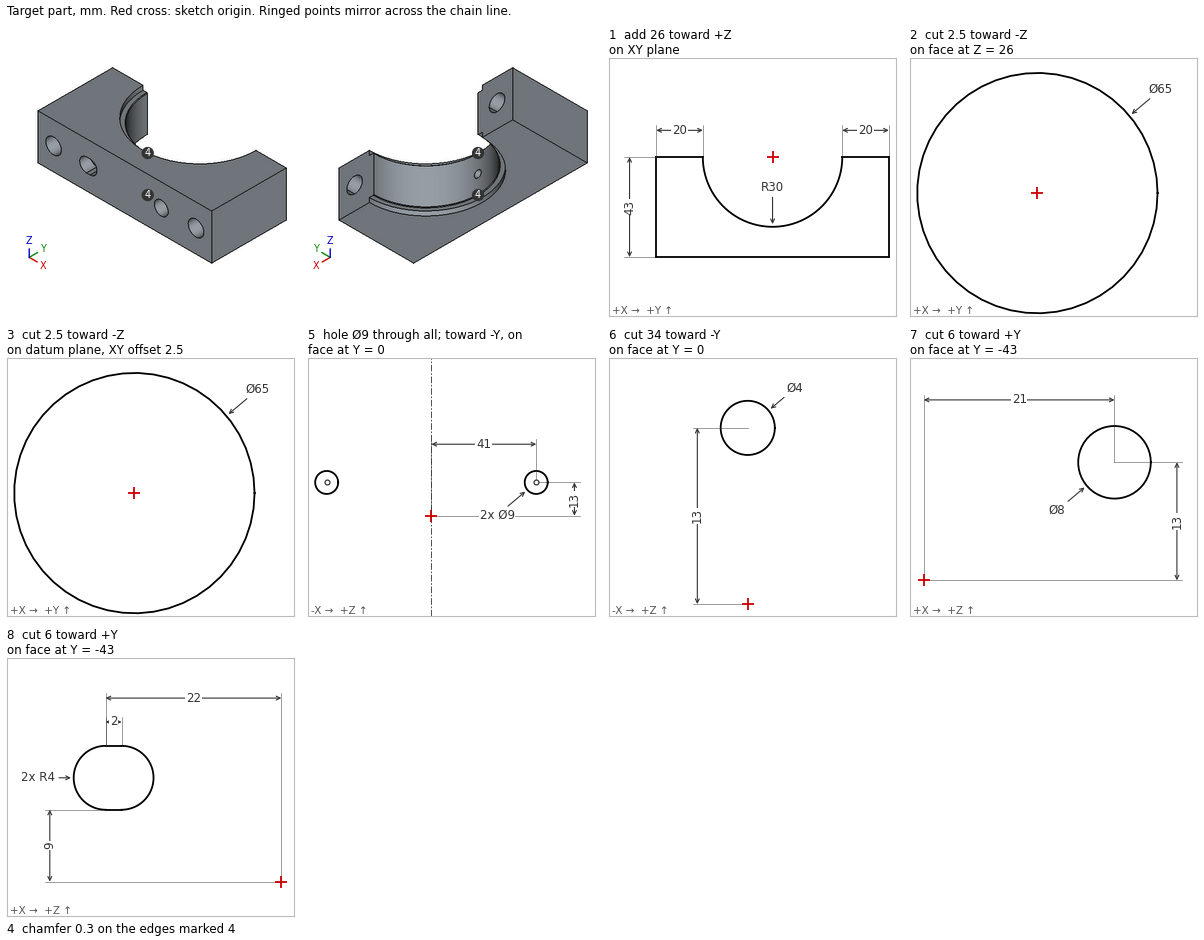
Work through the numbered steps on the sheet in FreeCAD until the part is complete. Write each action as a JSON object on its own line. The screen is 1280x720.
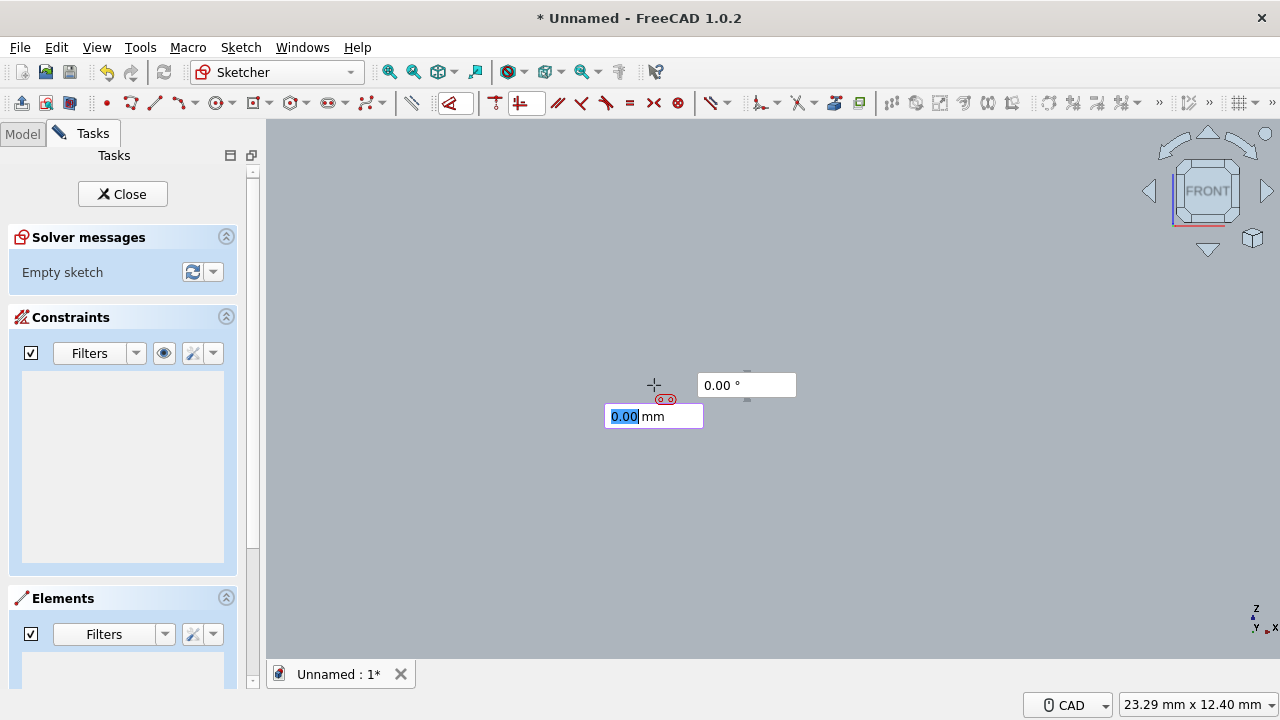
{"action": "left_click", "coordinate": [742, 385]}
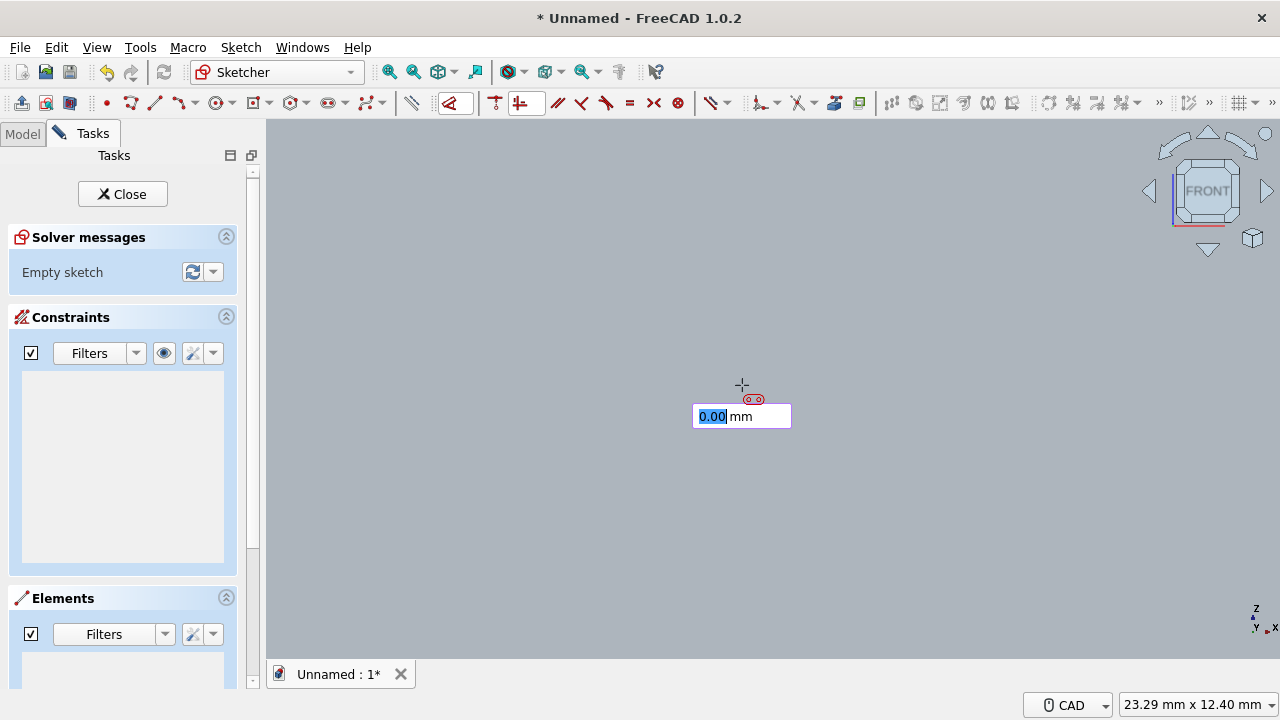
{"action": "left_click", "coordinate": [698, 211]}
{"action": "key", "text": "Escape"}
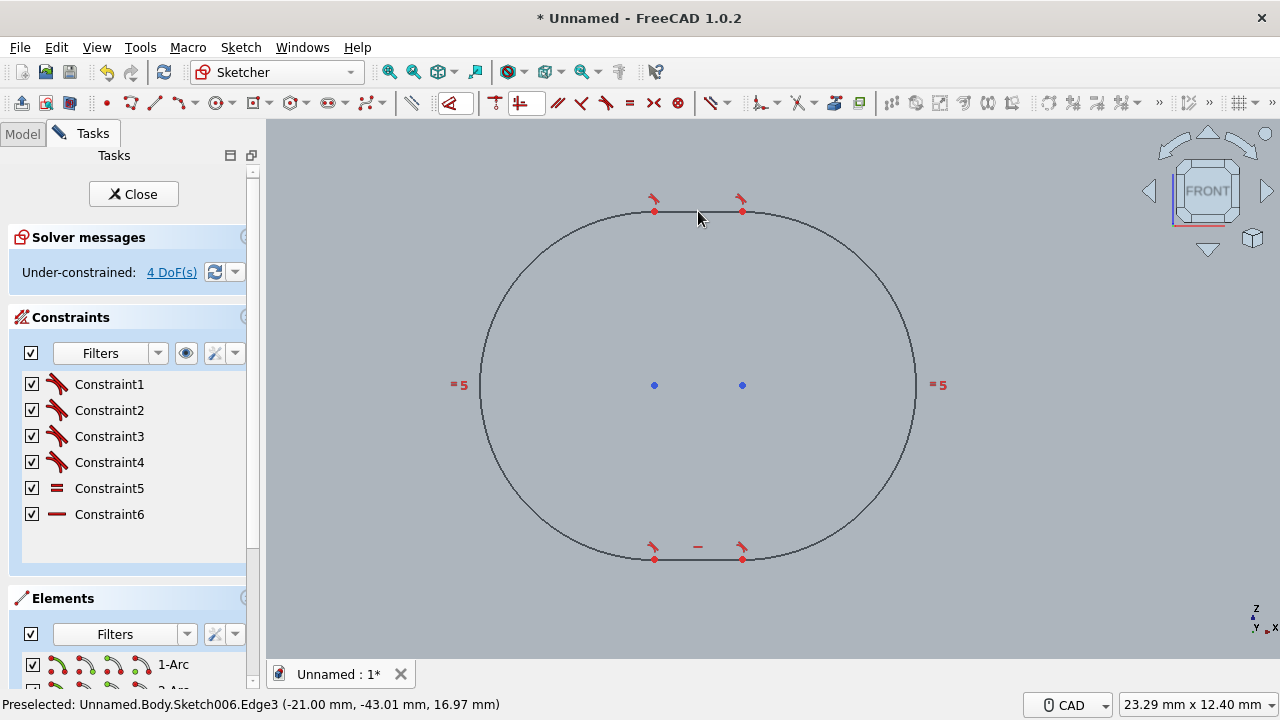
{"action": "left_click", "coordinate": [513, 284]}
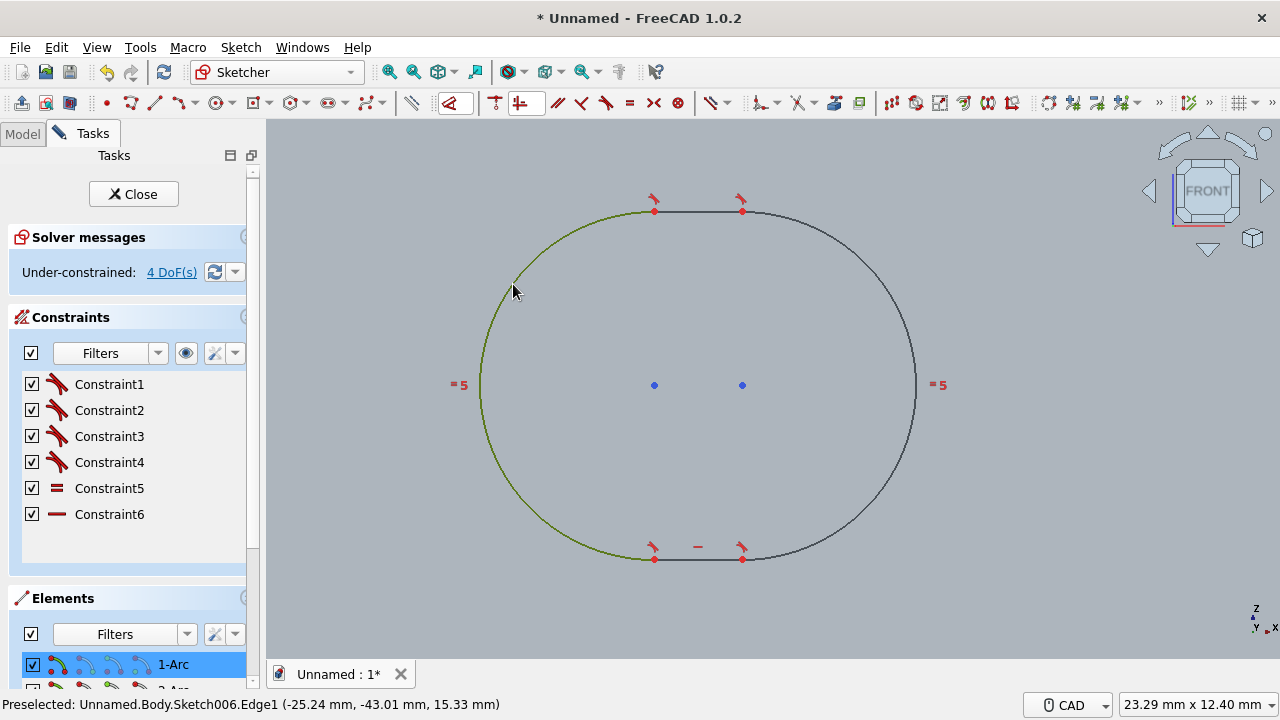
{"action": "left_click", "coordinate": [468, 104]}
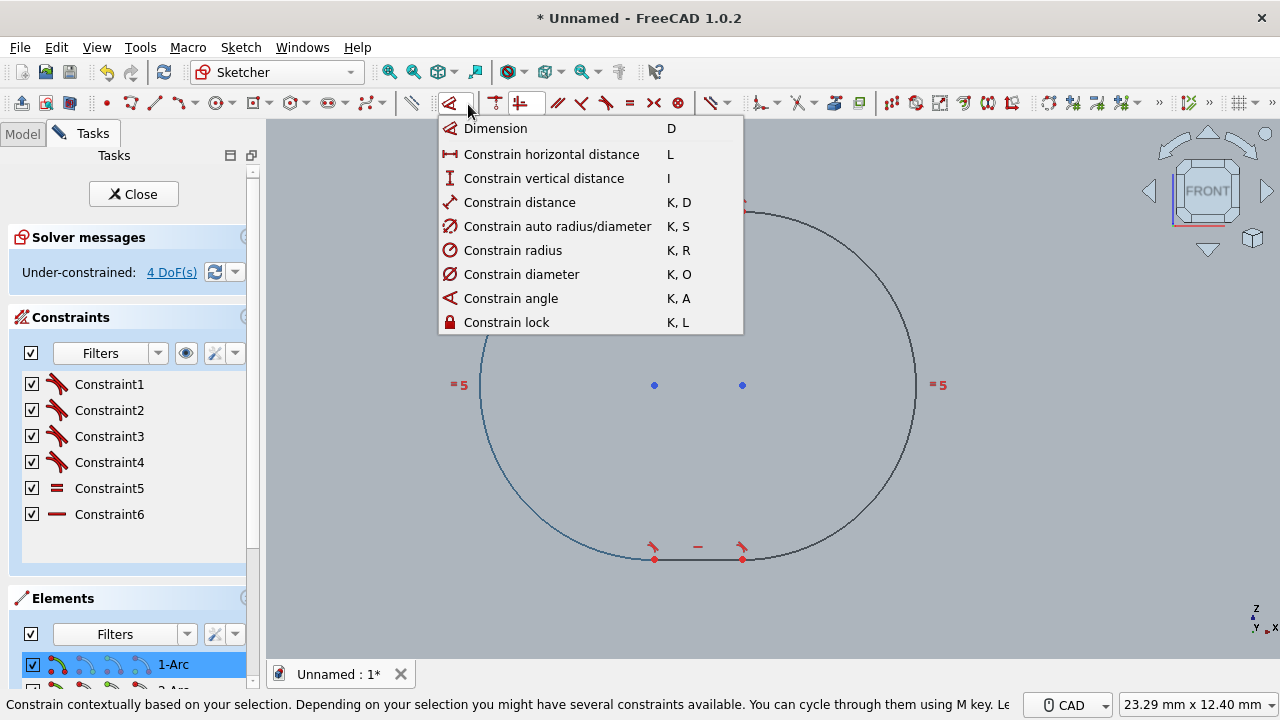
{"action": "left_click", "coordinate": [591, 250]}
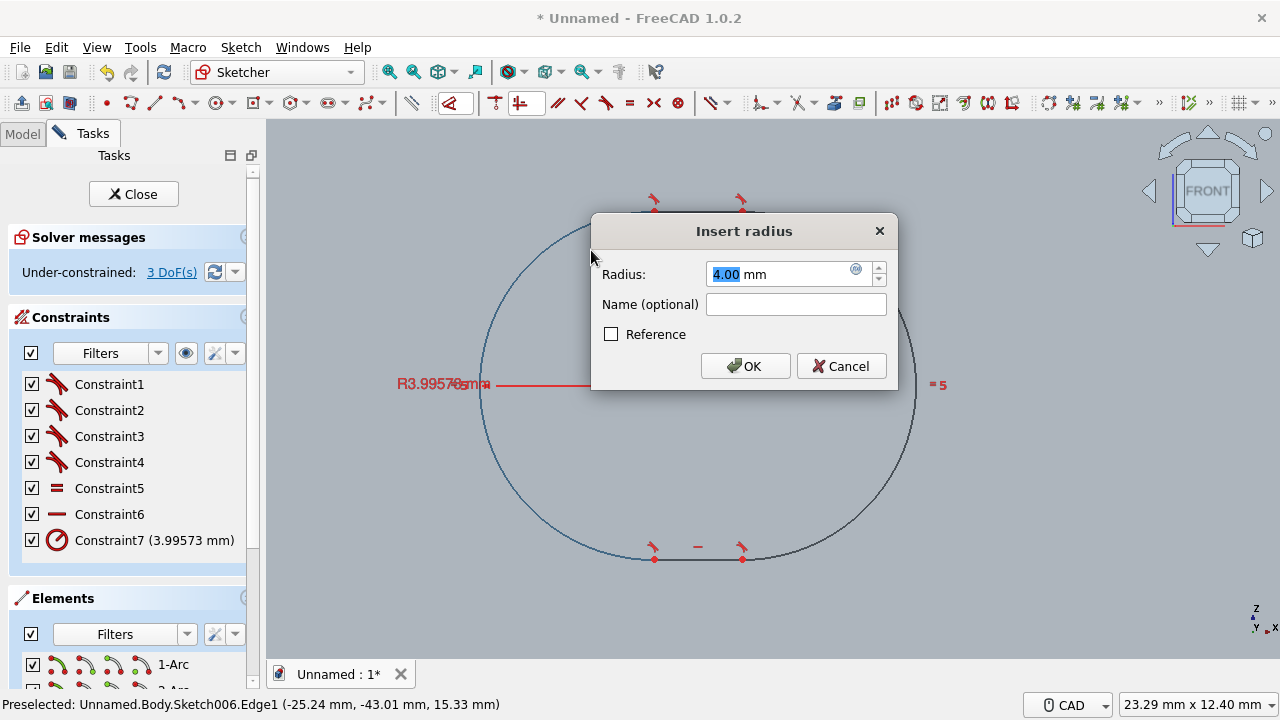
{"action": "type", "text": "4"}
{"action": "key", "text": "Return"}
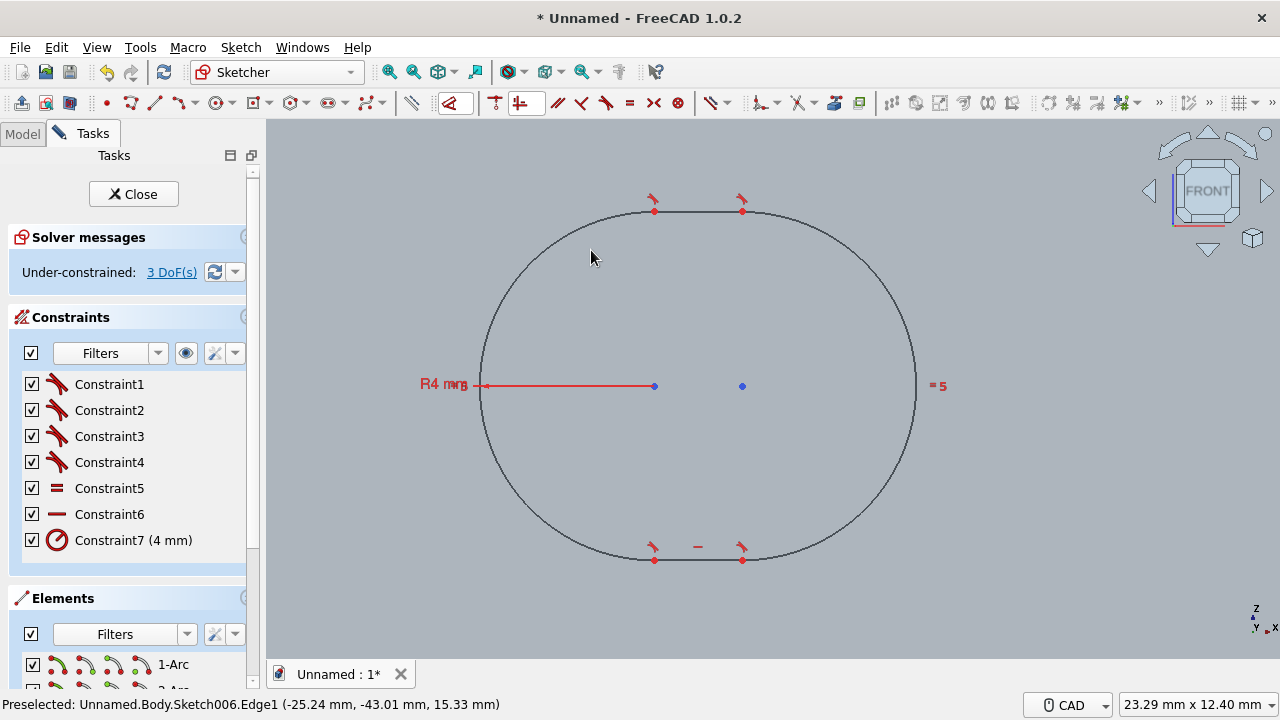
{"action": "left_click", "coordinate": [680, 212]}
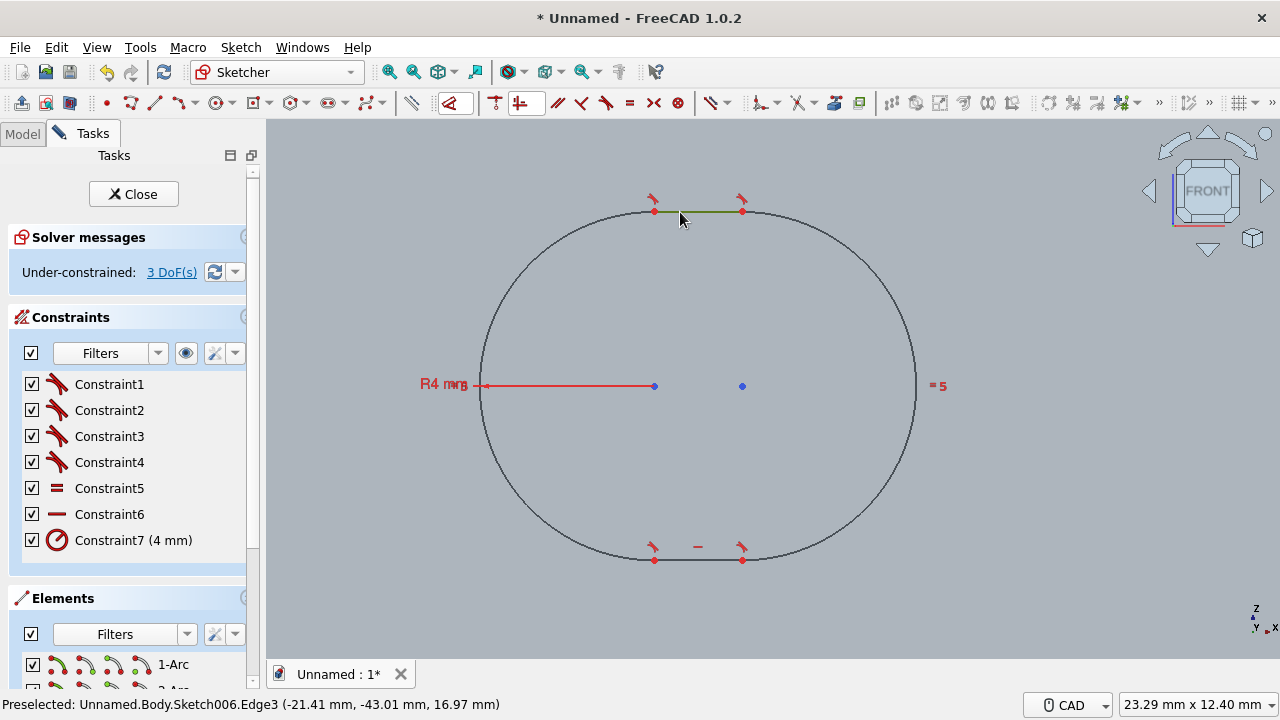
{"action": "left_click", "coordinate": [468, 104]}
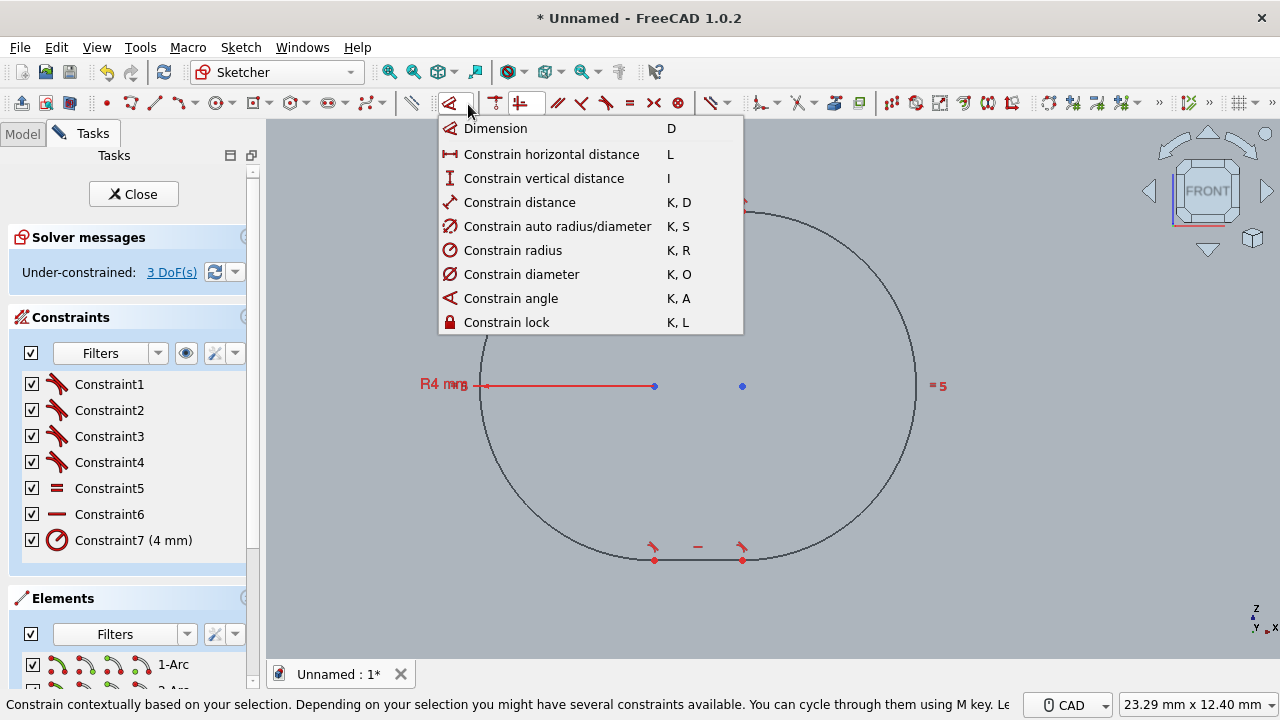
{"action": "left_click", "coordinate": [591, 154]}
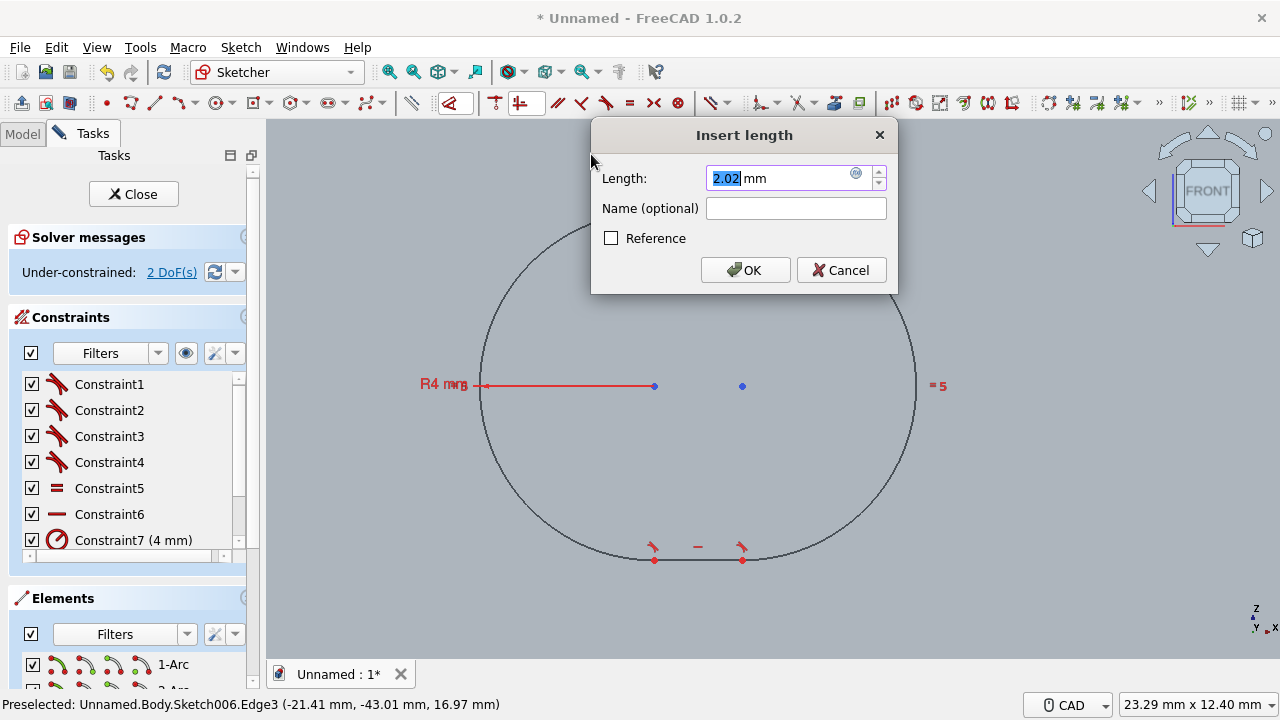
{"action": "type", "text": "2"}
{"action": "key", "text": "Return"}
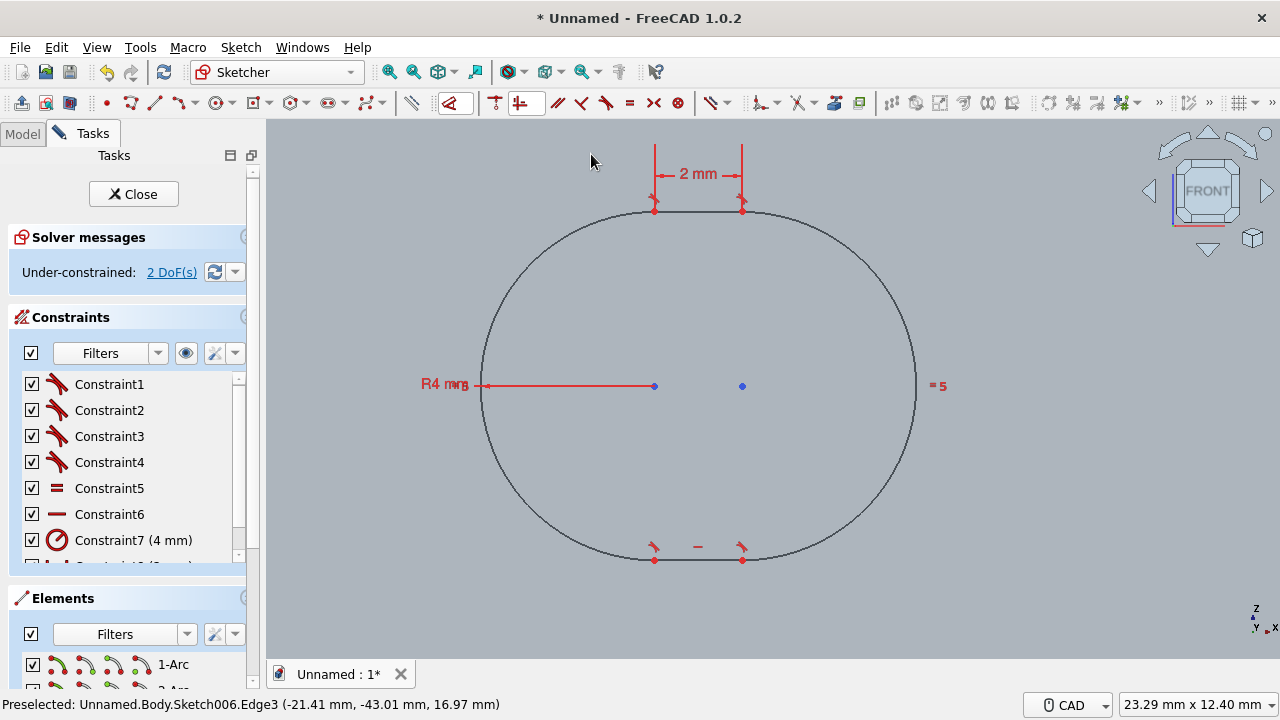
{"action": "left_click", "coordinate": [655, 560]}